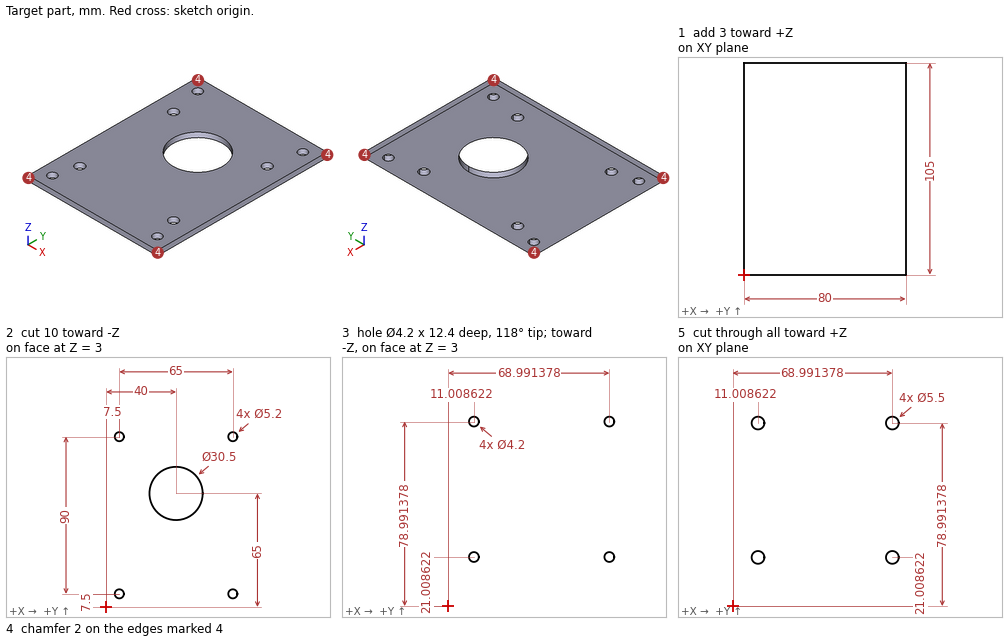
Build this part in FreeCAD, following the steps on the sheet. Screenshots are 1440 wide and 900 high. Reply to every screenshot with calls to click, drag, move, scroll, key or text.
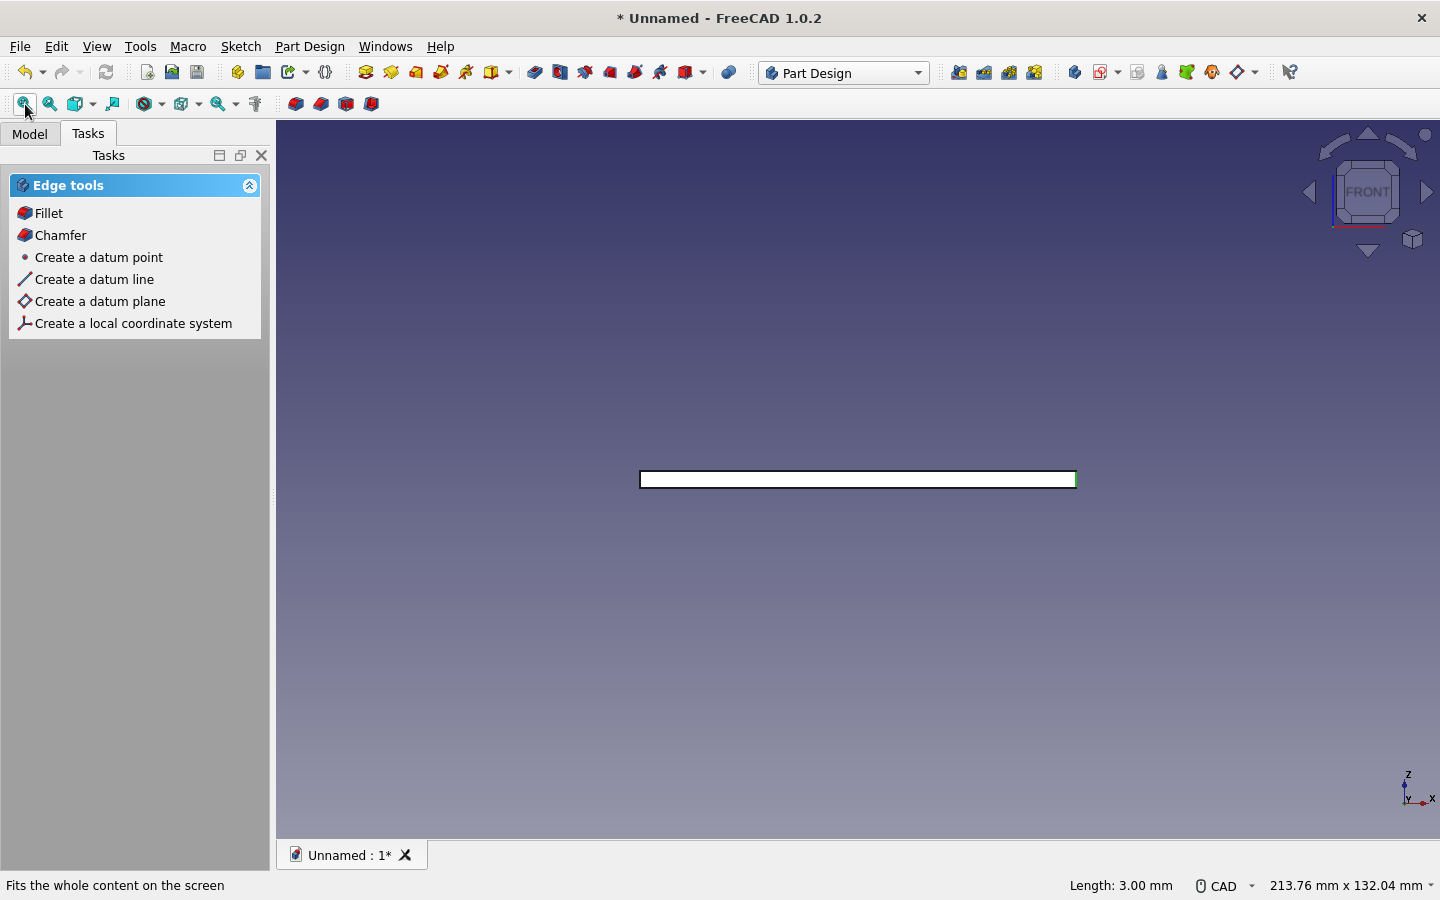
click(640, 479, ctrl)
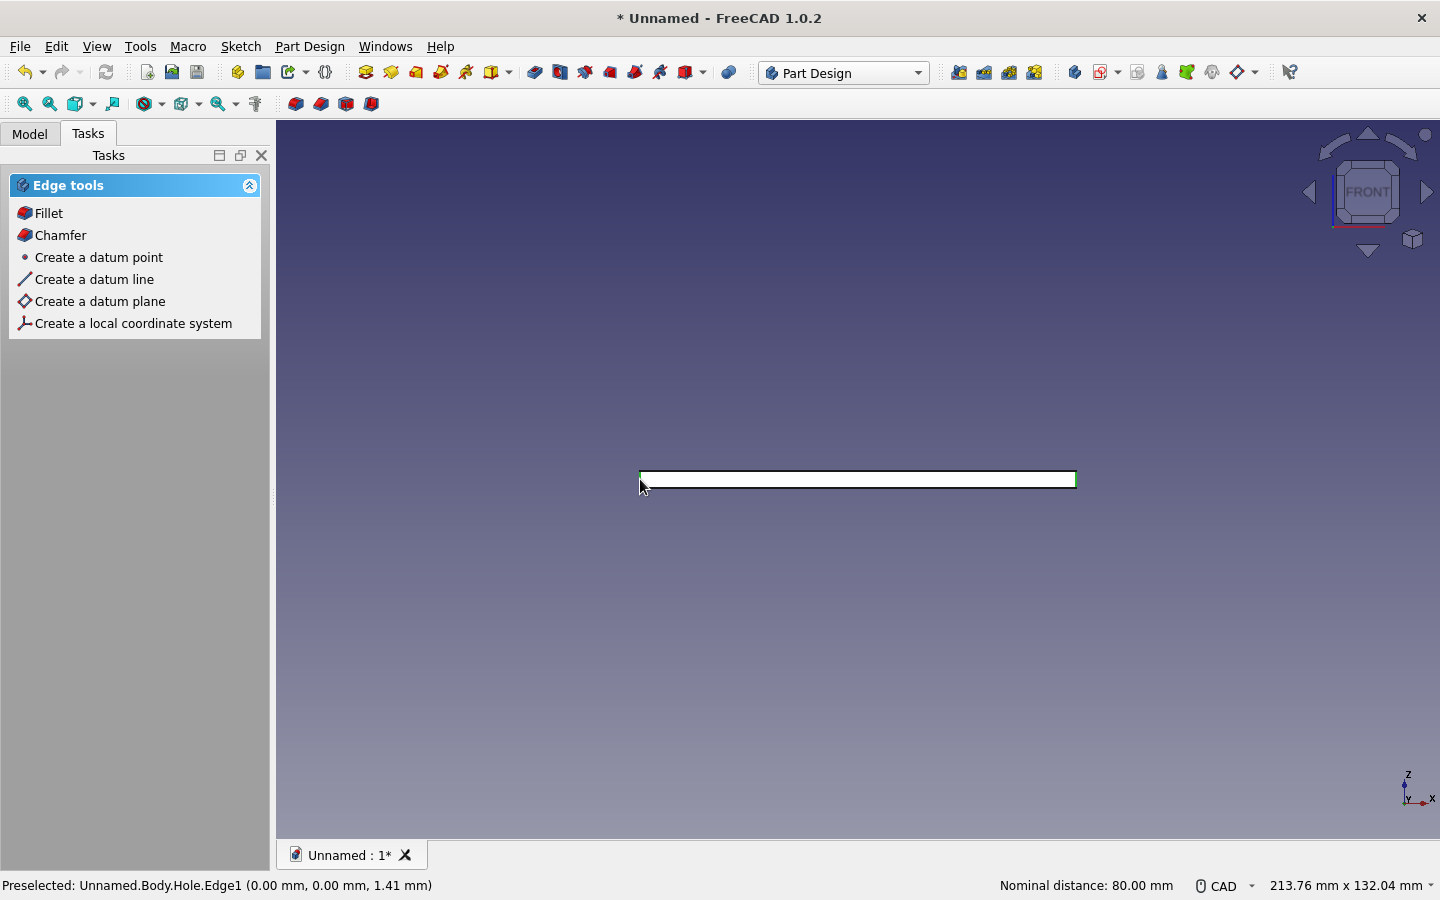
scroll(640, 479, up, 5)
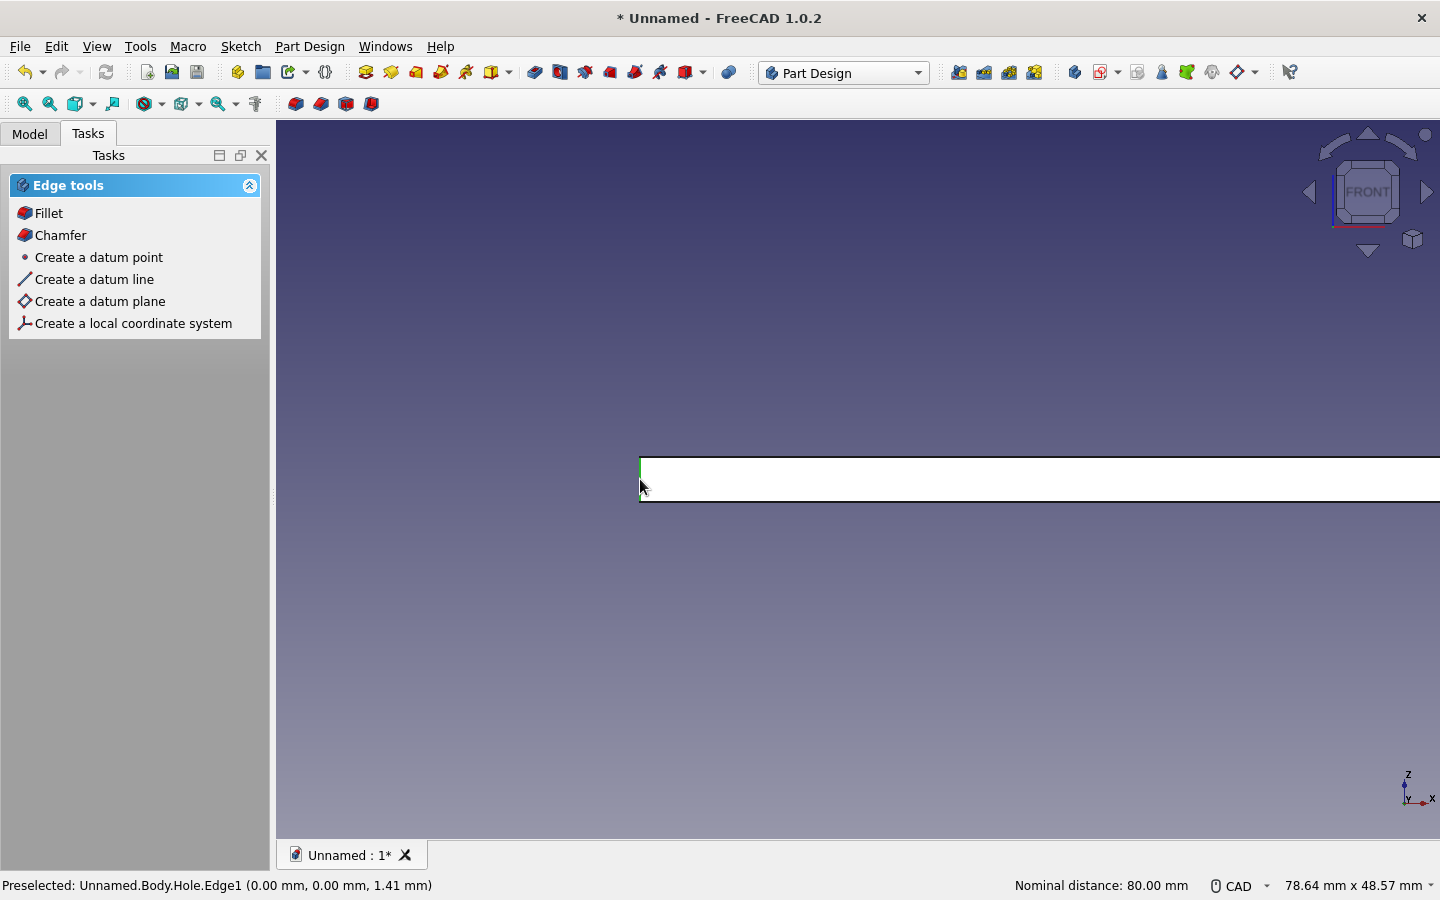
click(25, 104)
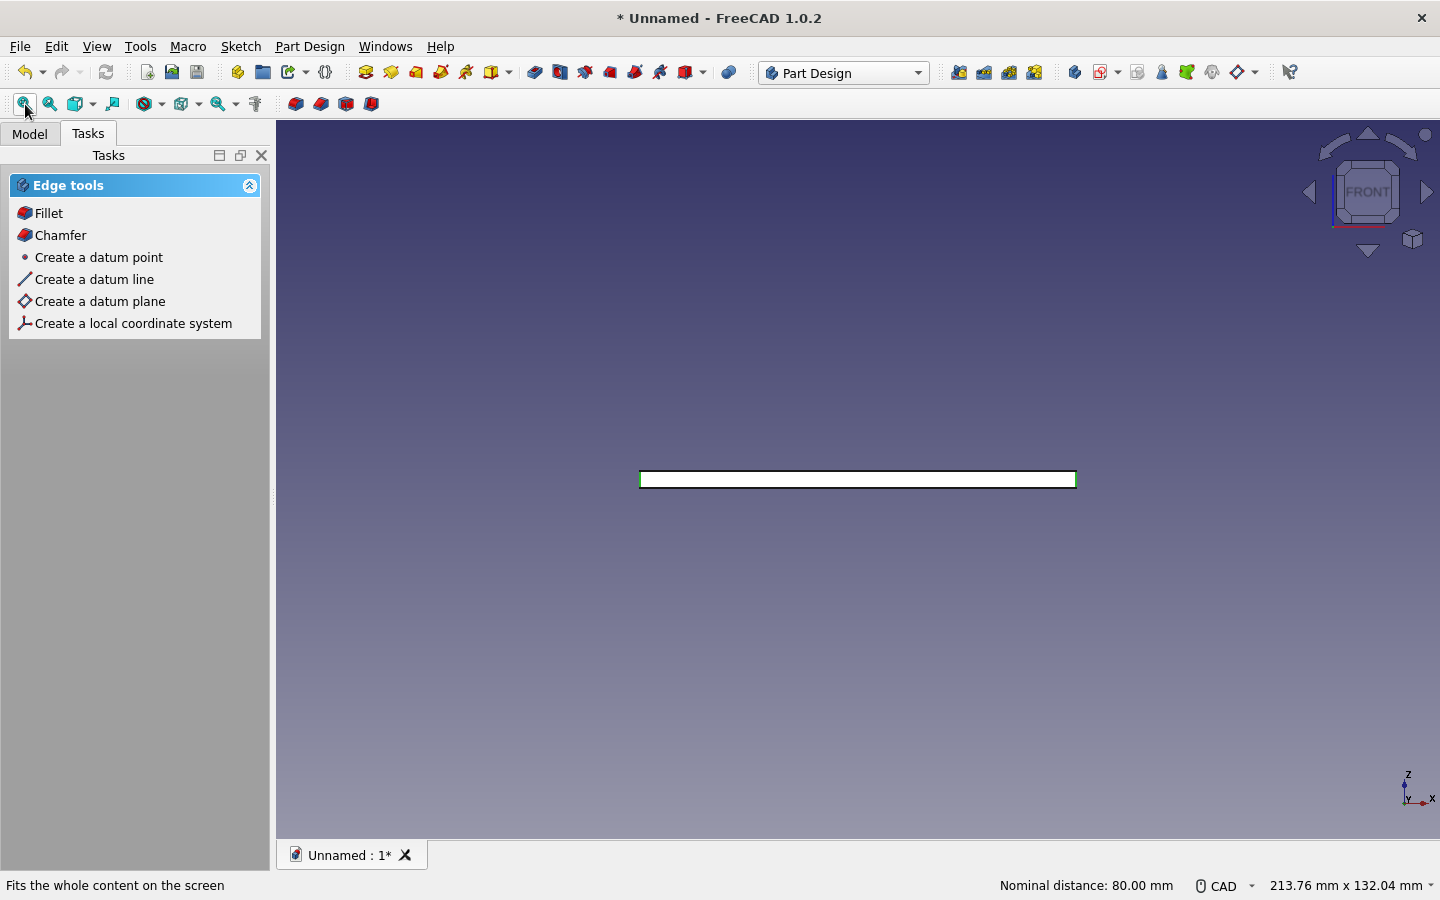
key(3)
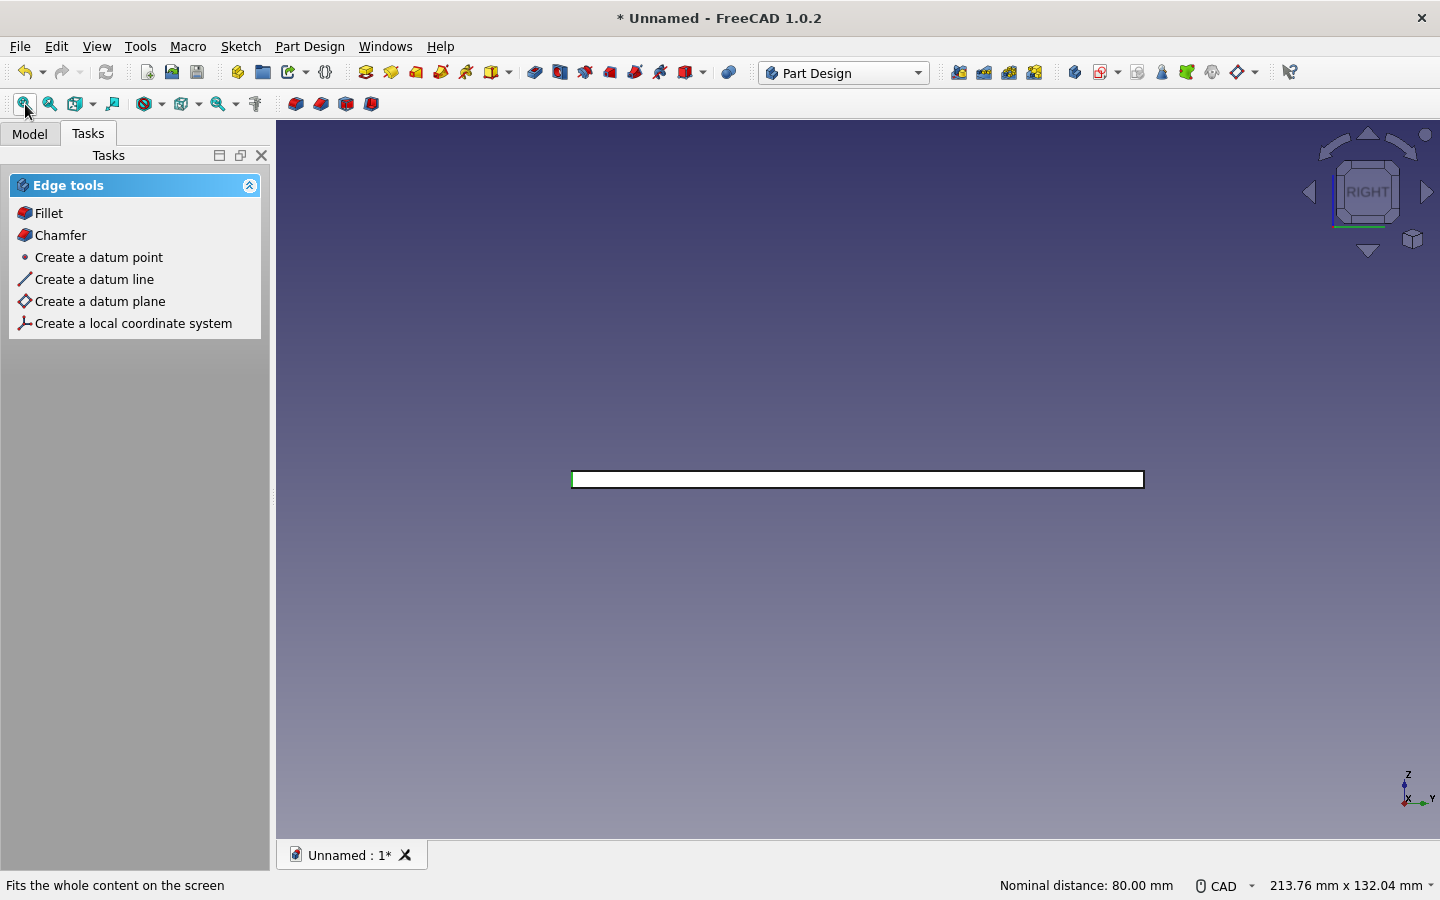
click(1144, 478, ctrl)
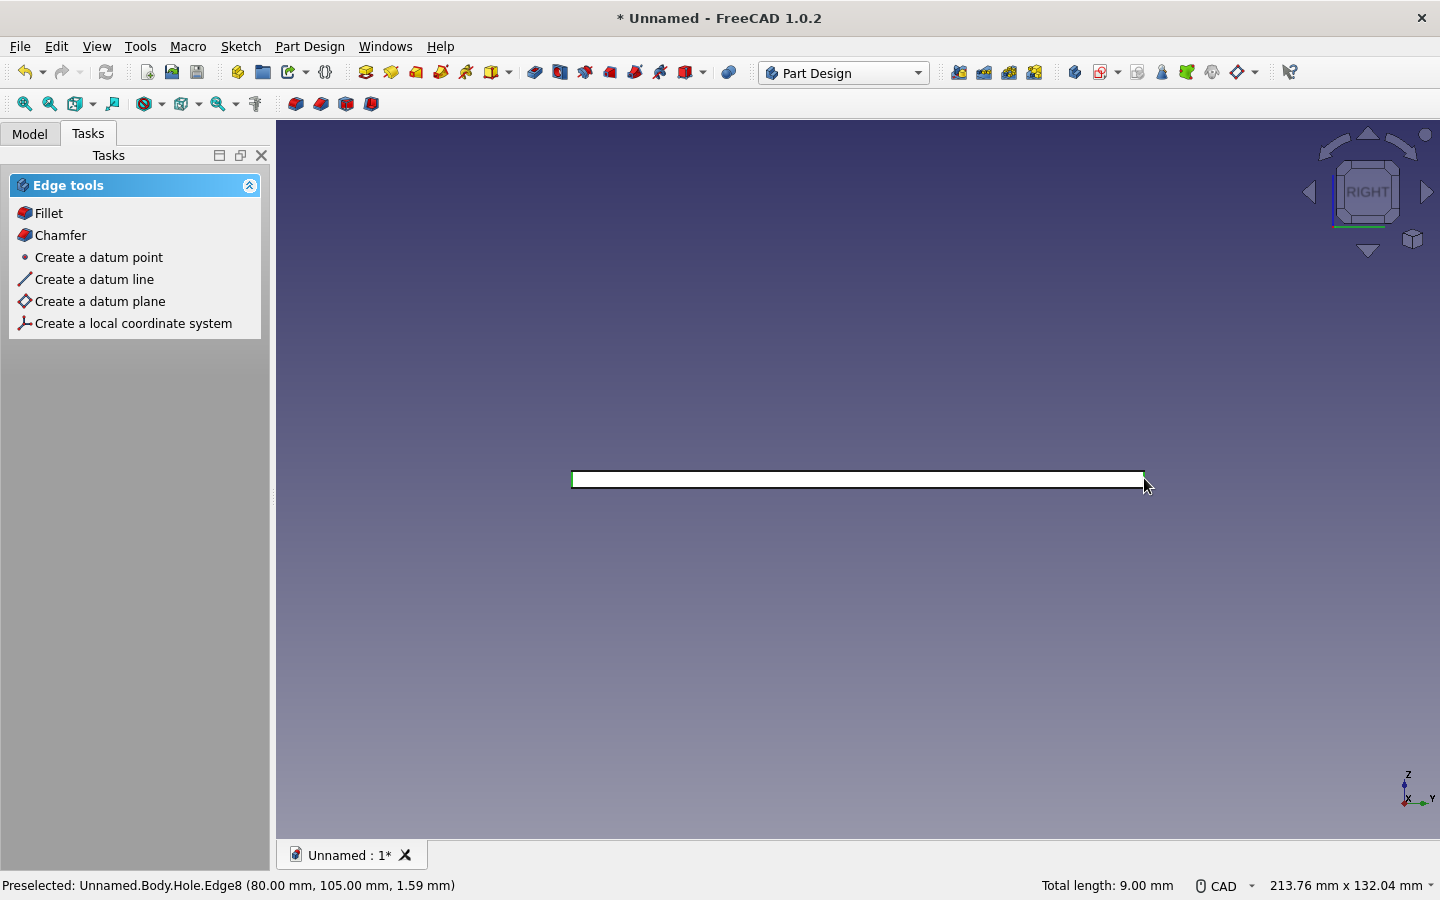
scroll(1144, 478, up, 5)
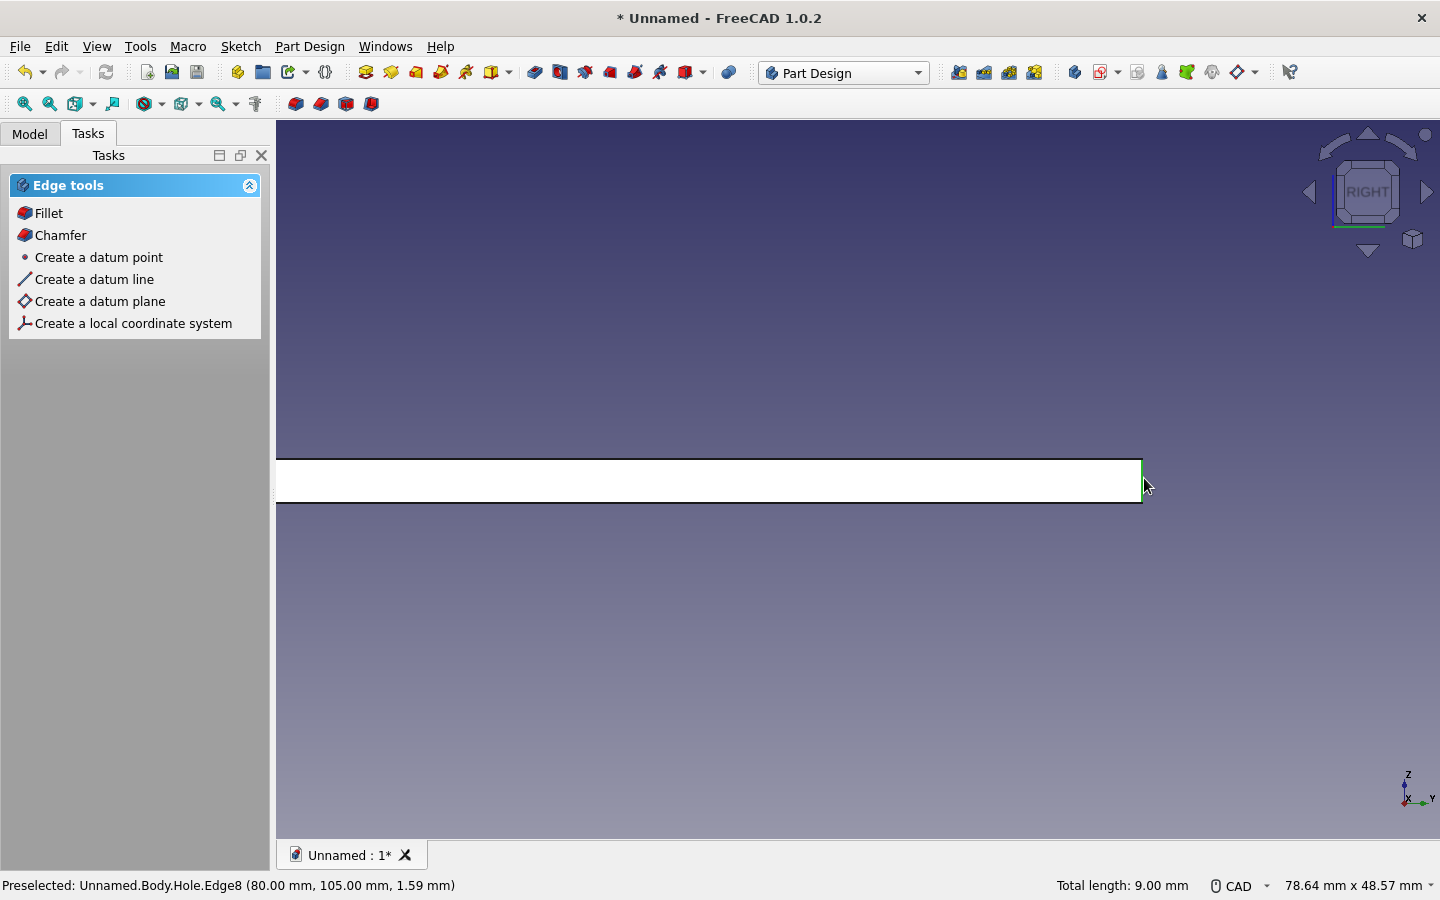
click(25, 104)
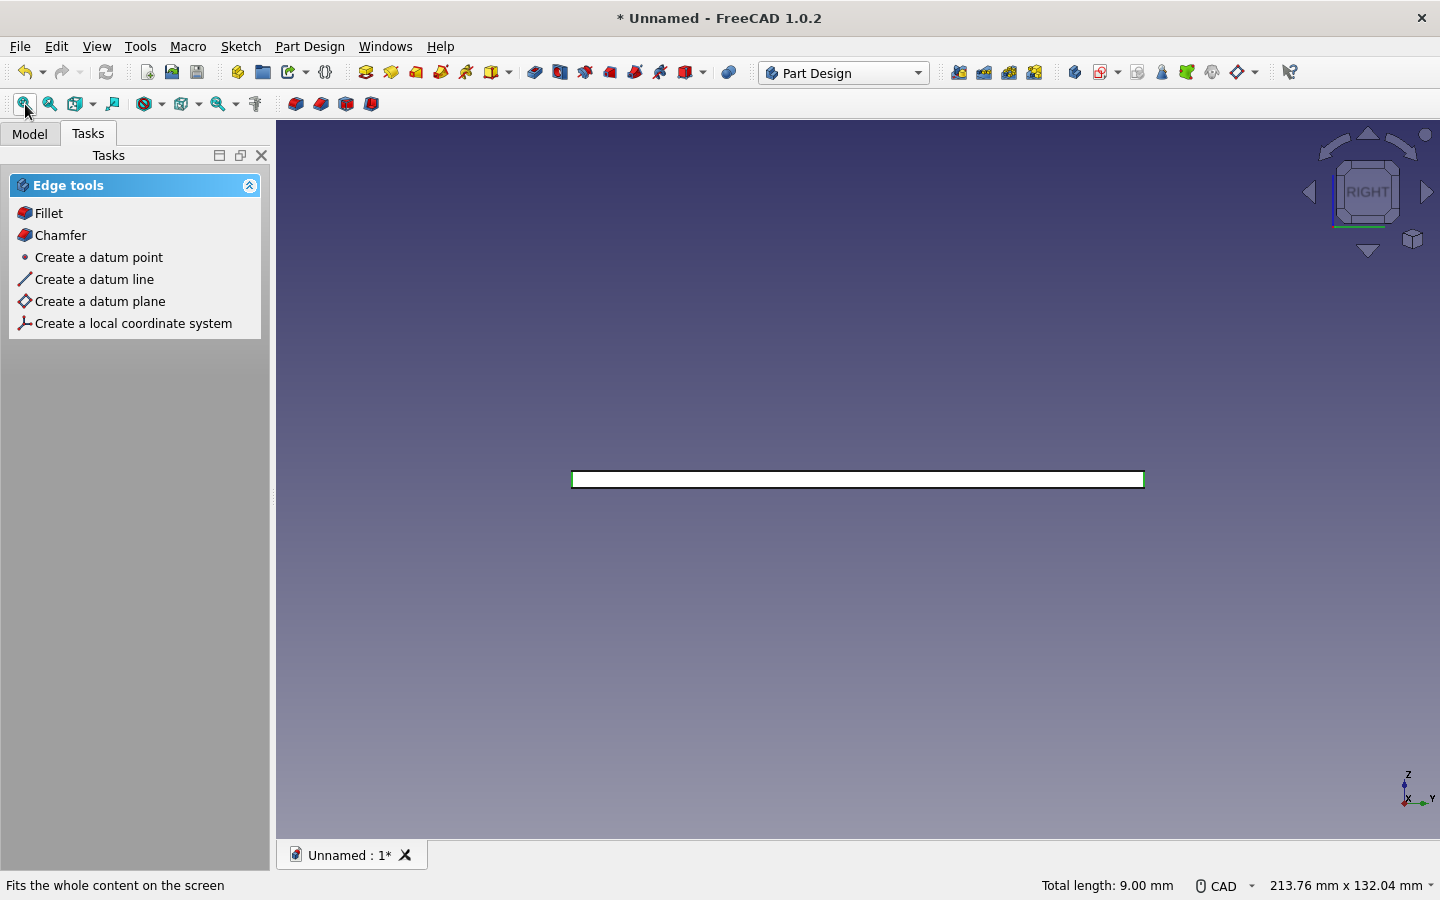
key(5)